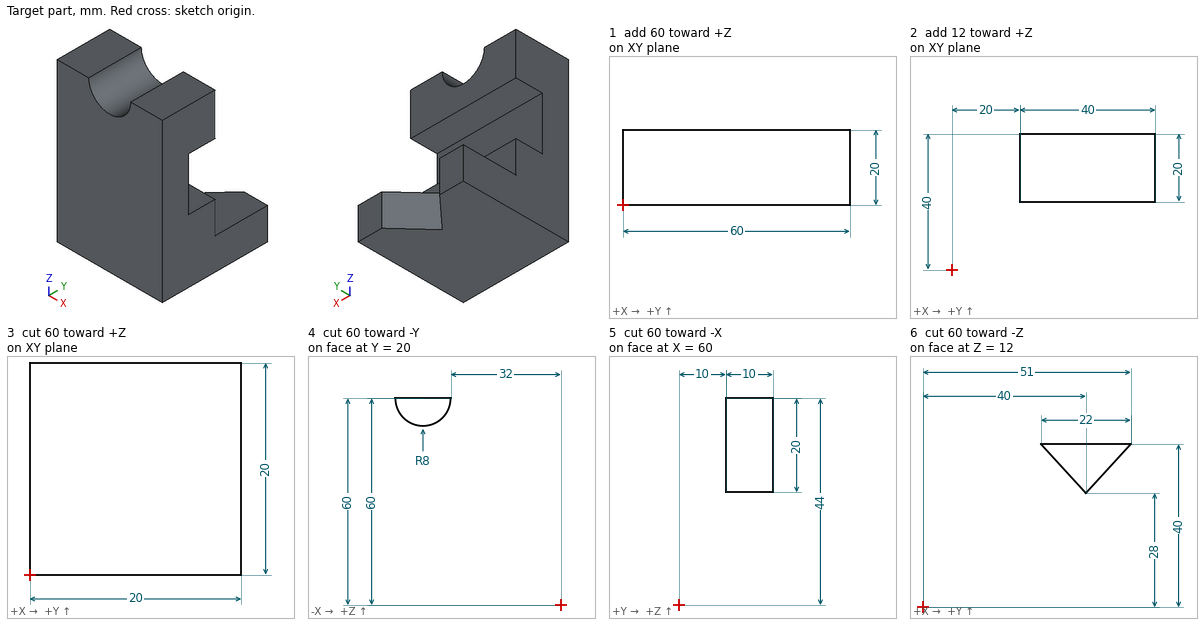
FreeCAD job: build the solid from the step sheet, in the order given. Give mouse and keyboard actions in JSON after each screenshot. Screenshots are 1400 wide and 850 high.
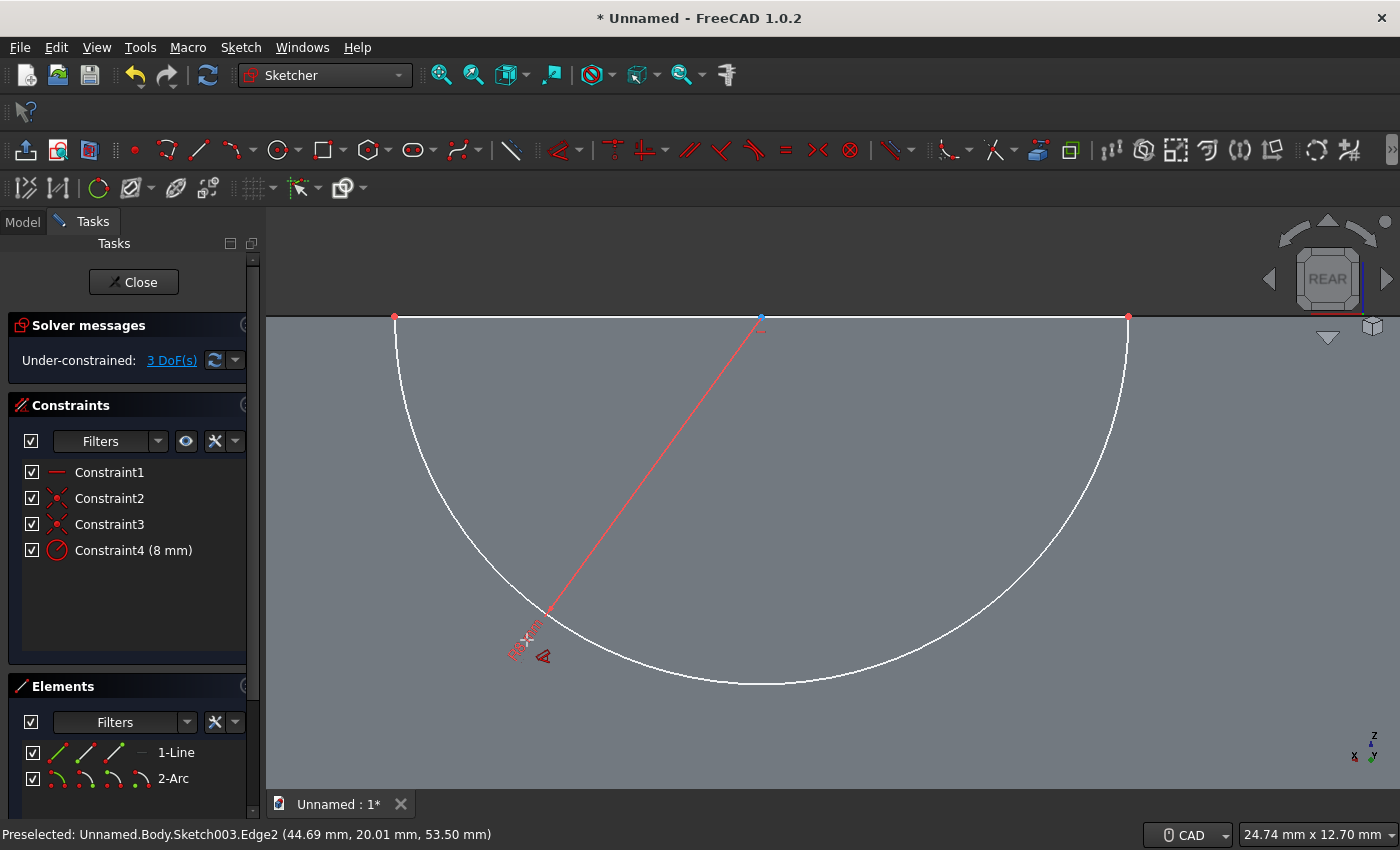
{"action": "left_click", "coordinate": [1128, 317]}
{"action": "left_click", "coordinate": [1182, 283]}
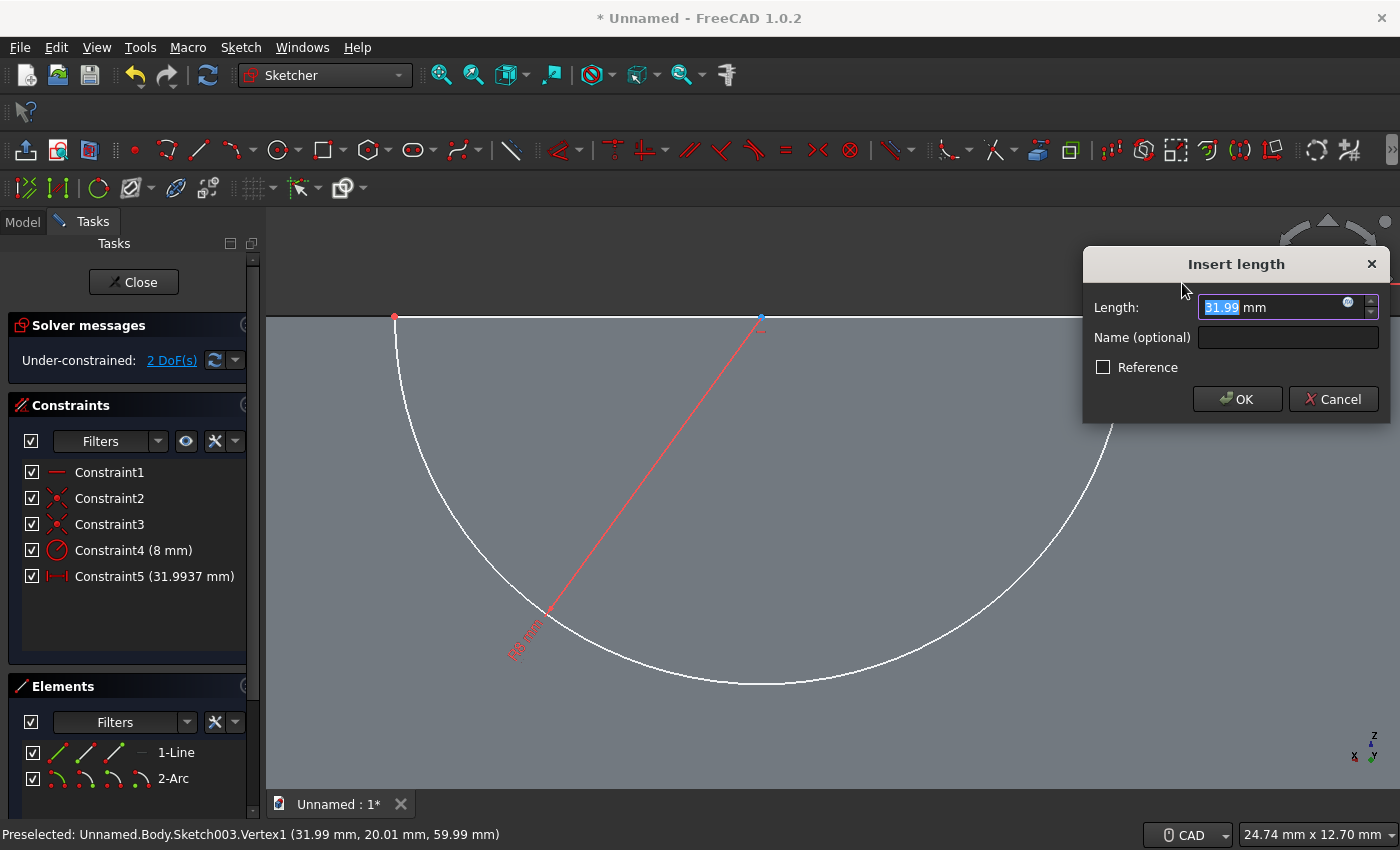
{"action": "type", "text": "32"}
{"action": "key", "text": "Return"}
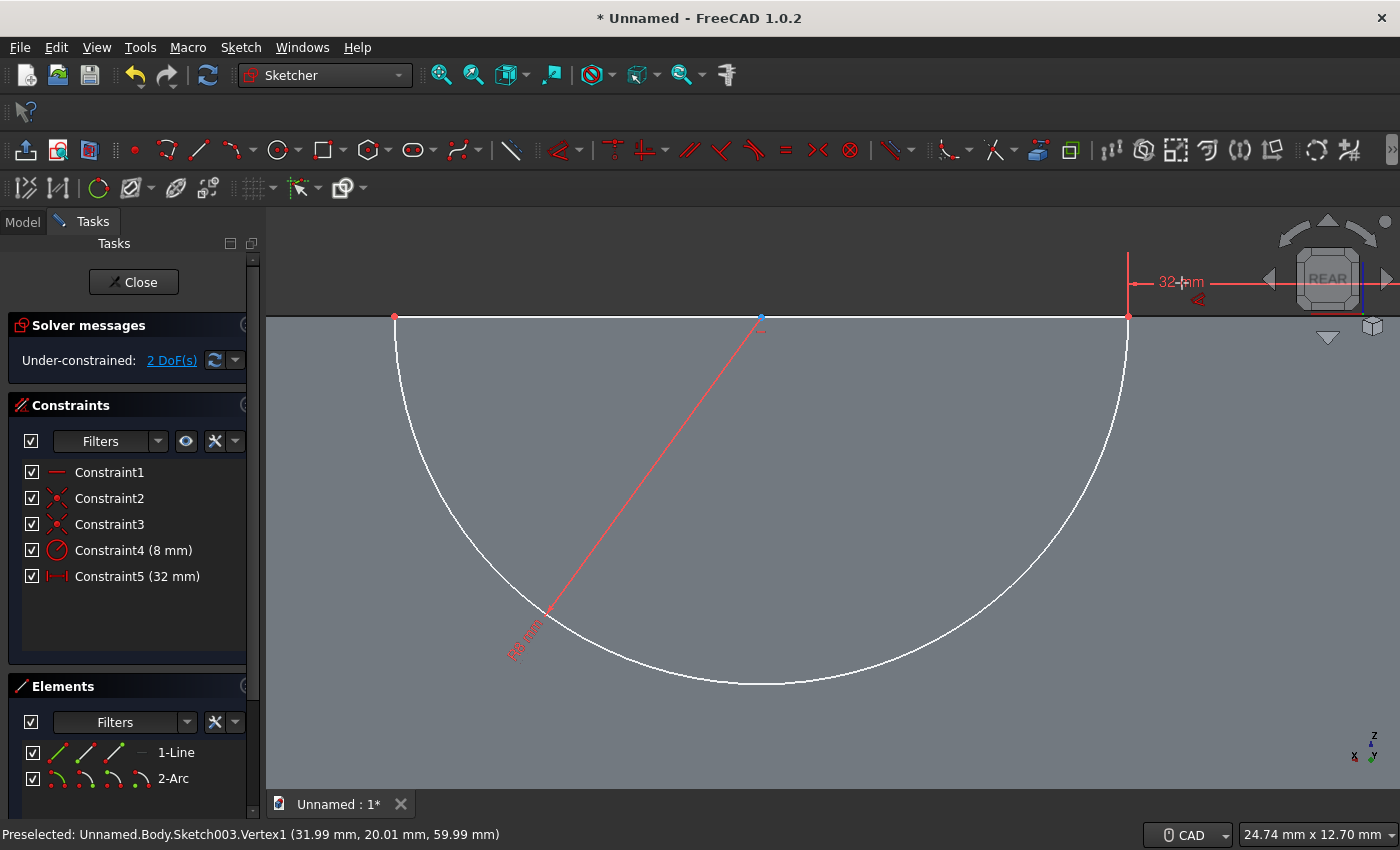
{"action": "left_click", "coordinate": [1128, 317]}
{"action": "left_click", "coordinate": [1094, 539]}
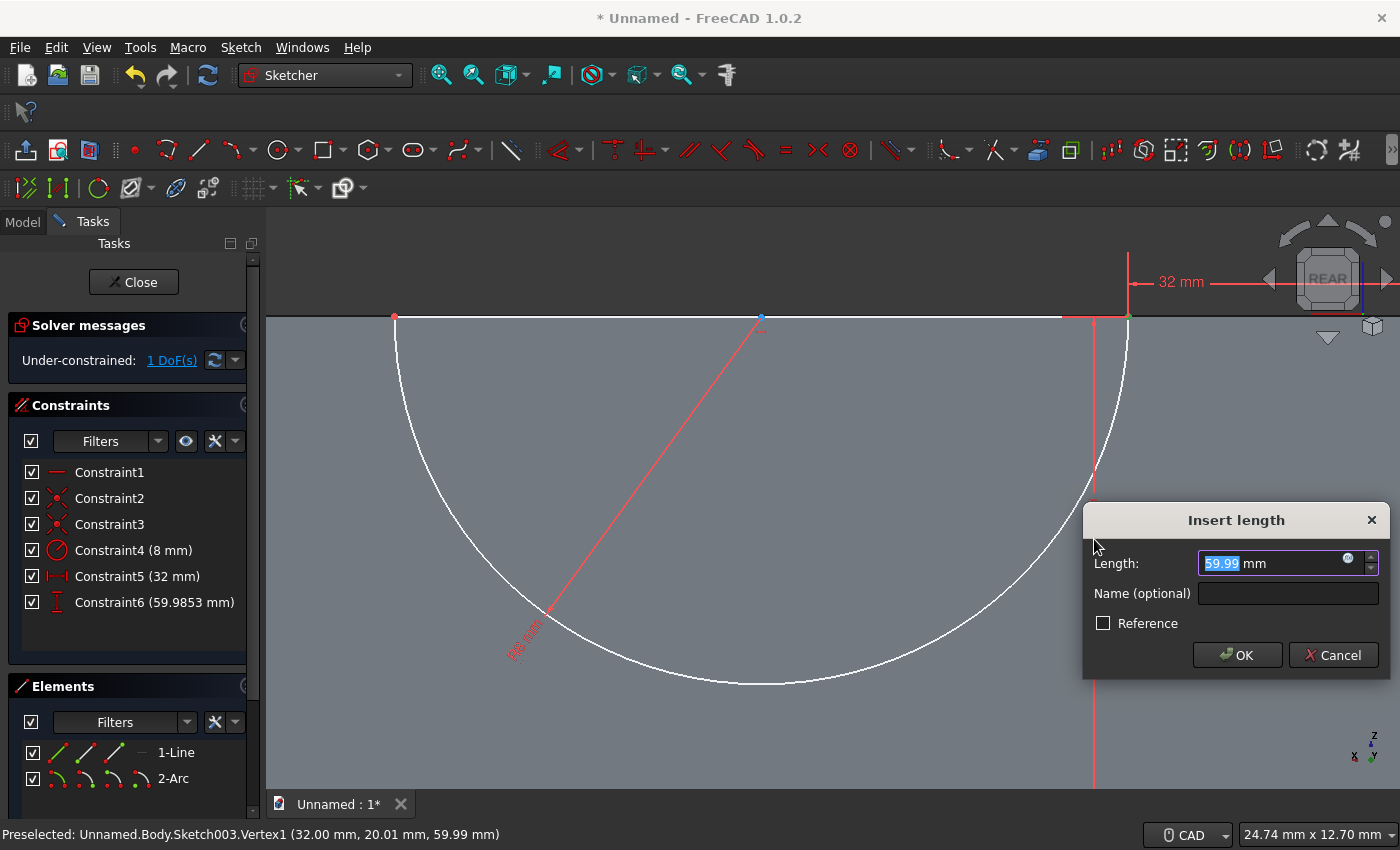
{"action": "type", "text": "60"}
{"action": "key", "text": "Return"}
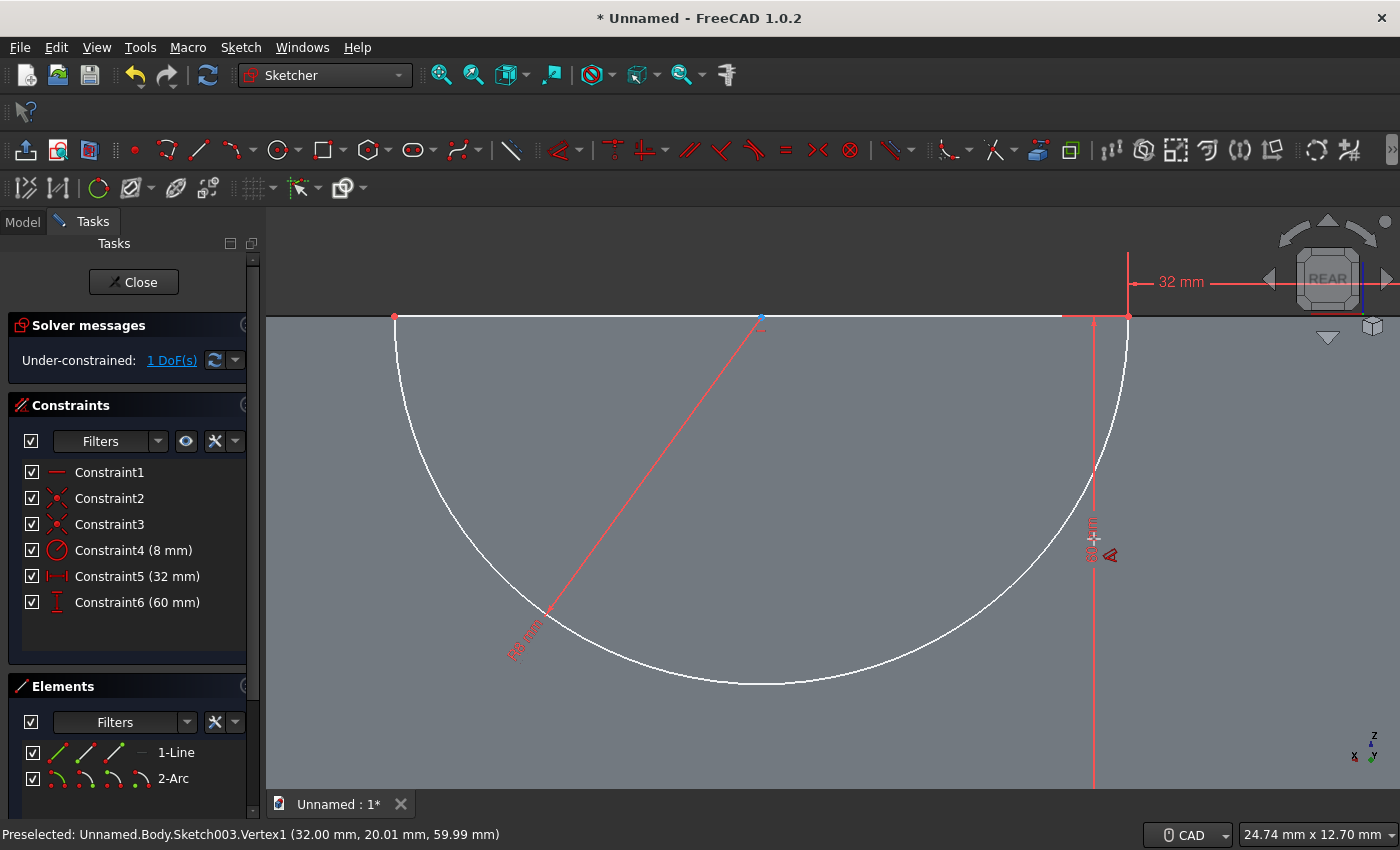
{"action": "left_click", "coordinate": [761, 317]}
{"action": "left_click", "coordinate": [727, 539]}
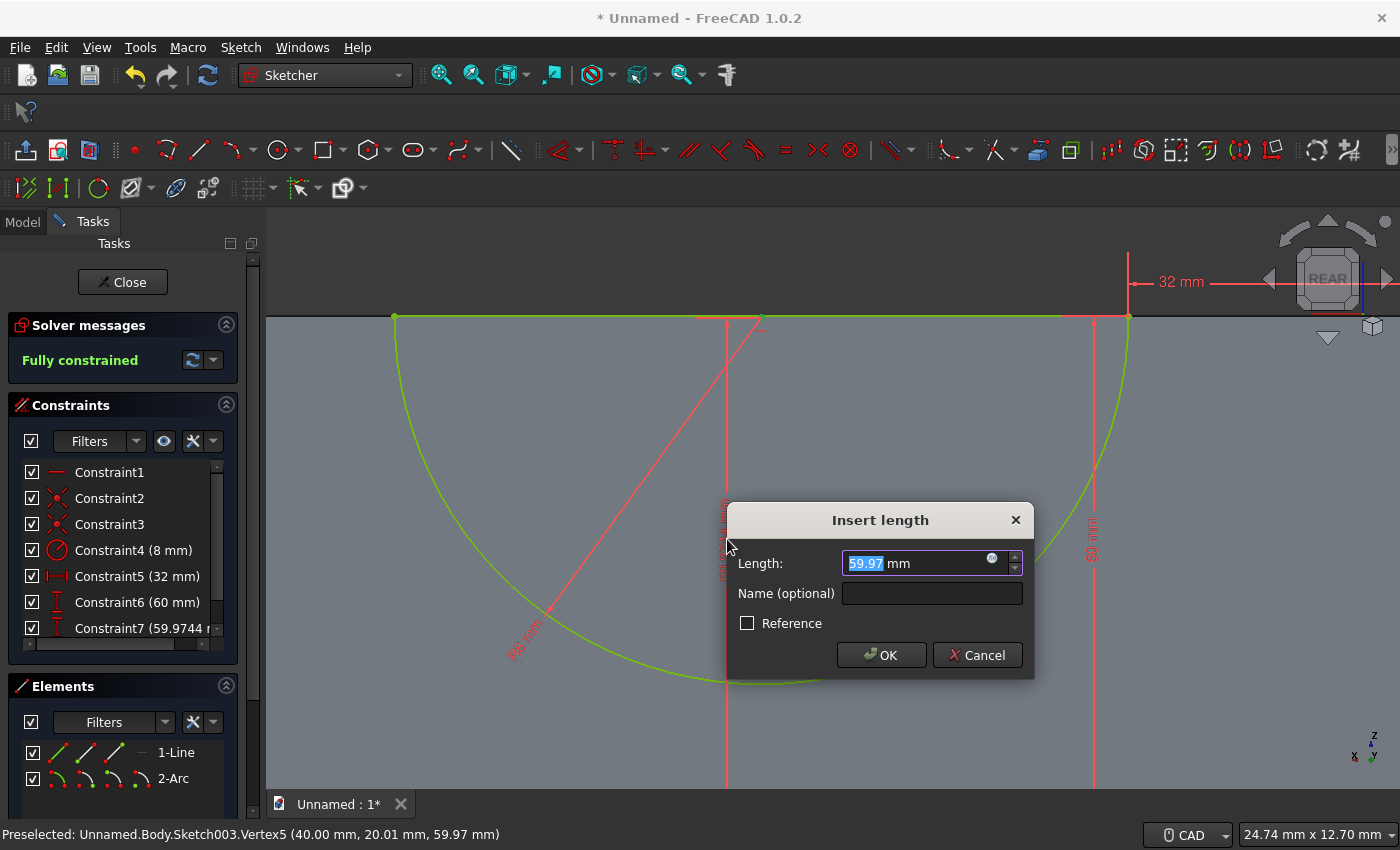
{"action": "type", "text": "60"}
{"action": "key", "text": "Return"}
{"action": "key", "text": "Escape"}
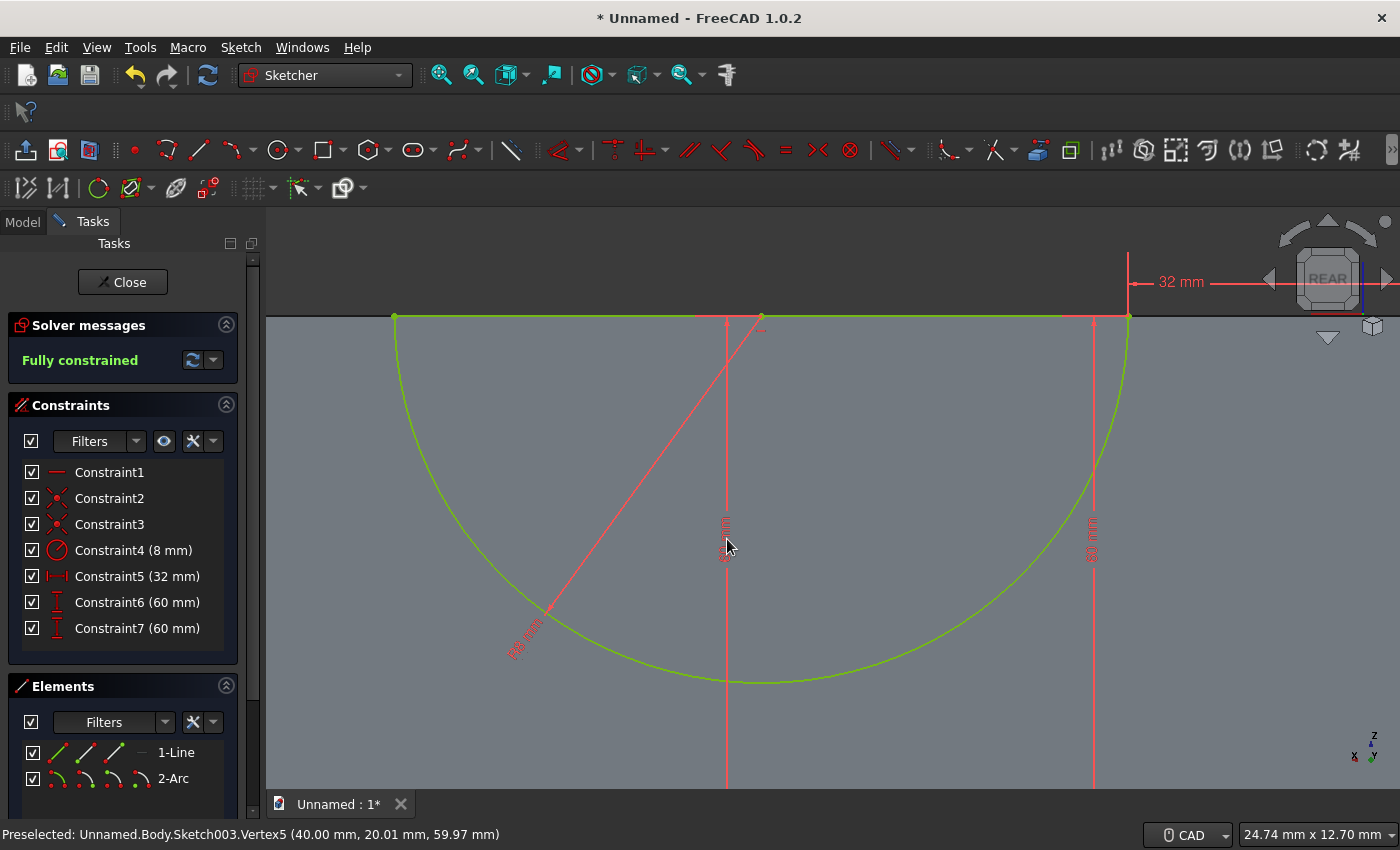
{"action": "left_click", "coordinate": [123, 282]}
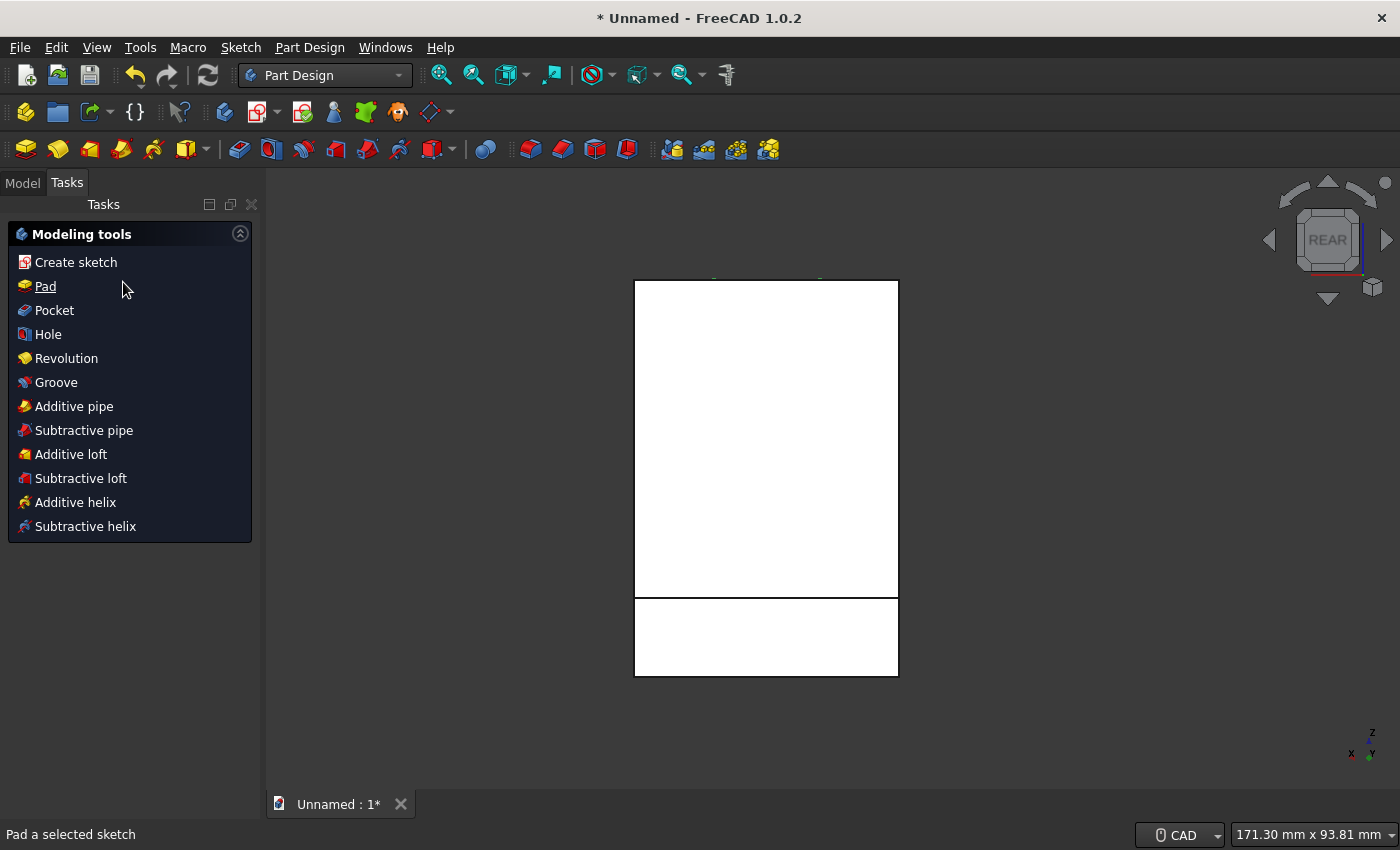
{"action": "left_click", "coordinate": [240, 150]}